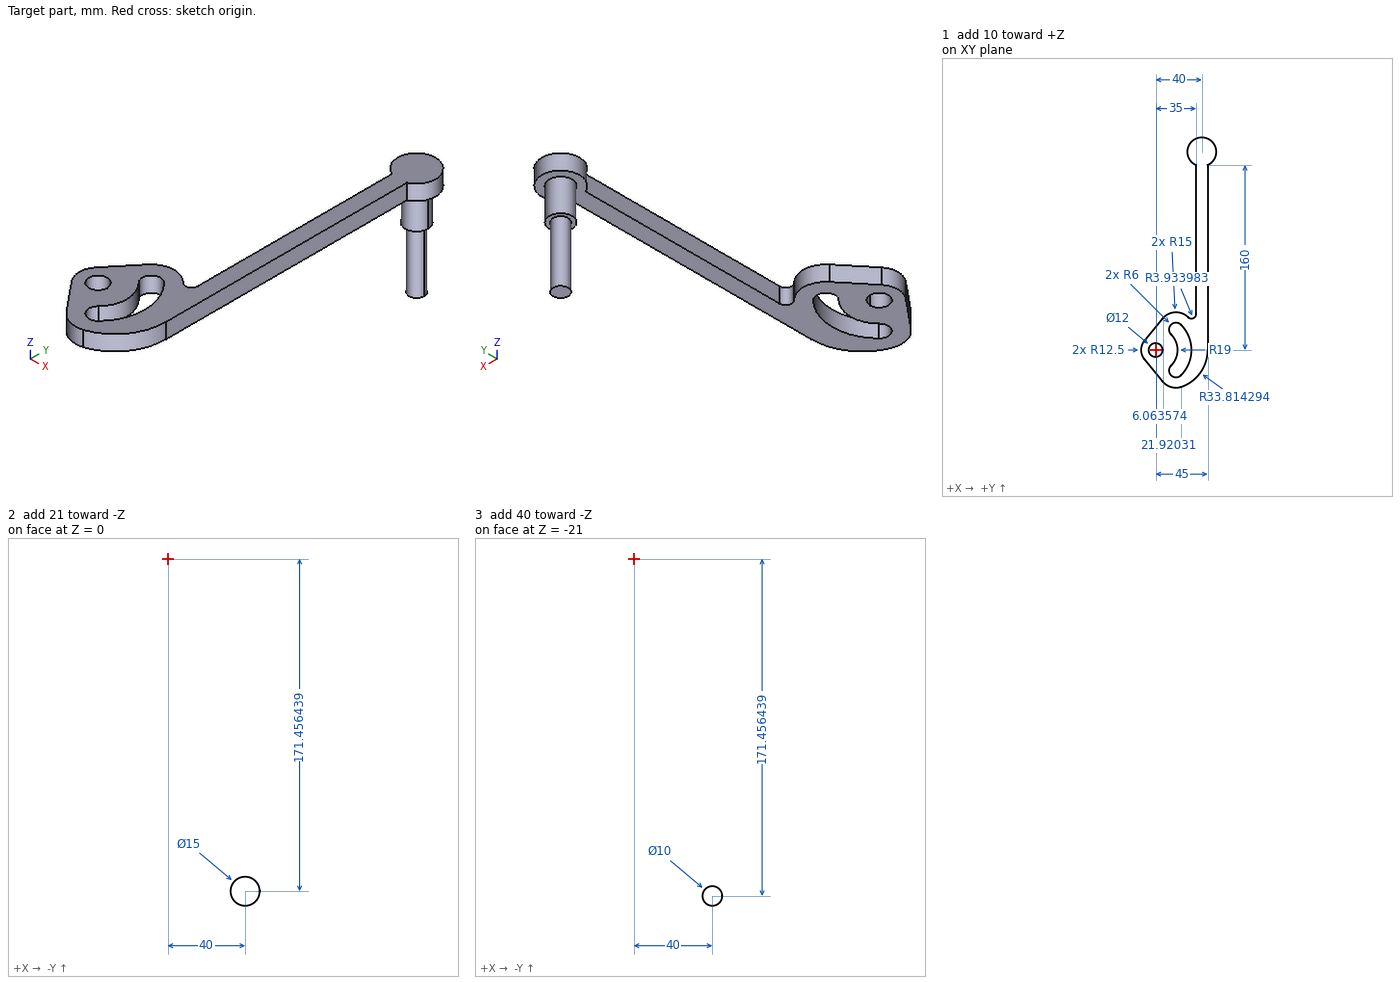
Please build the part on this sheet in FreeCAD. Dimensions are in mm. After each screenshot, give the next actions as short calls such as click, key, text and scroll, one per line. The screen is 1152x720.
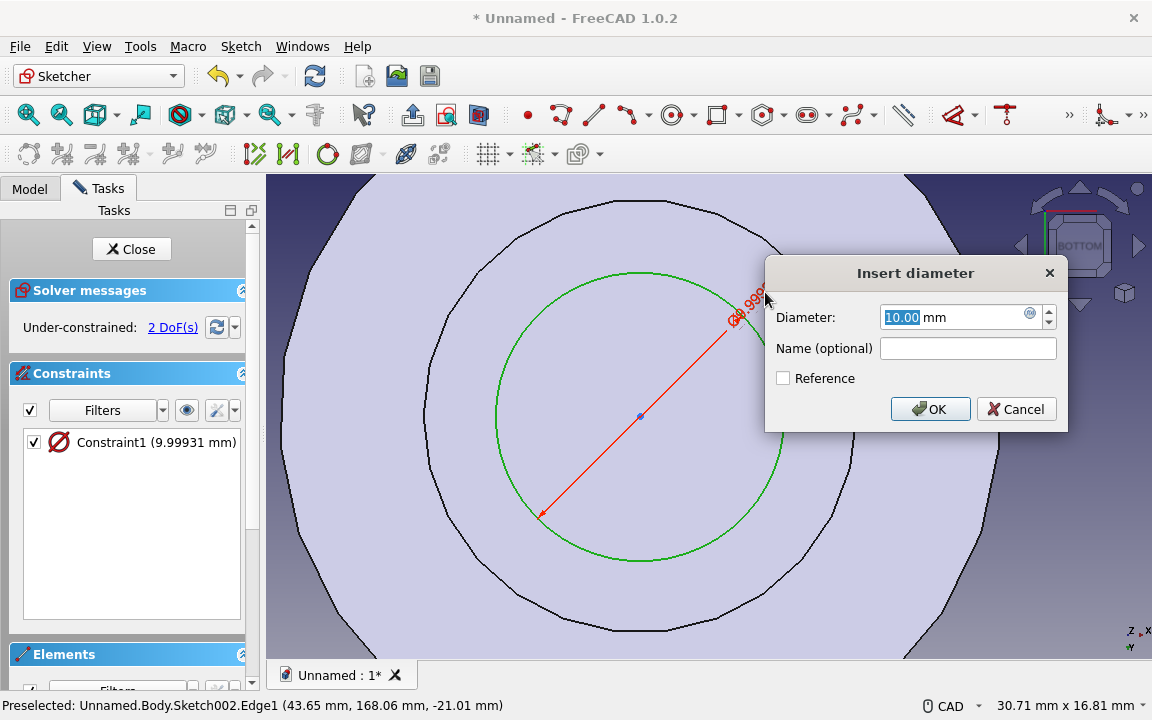
text(10)
key(Return)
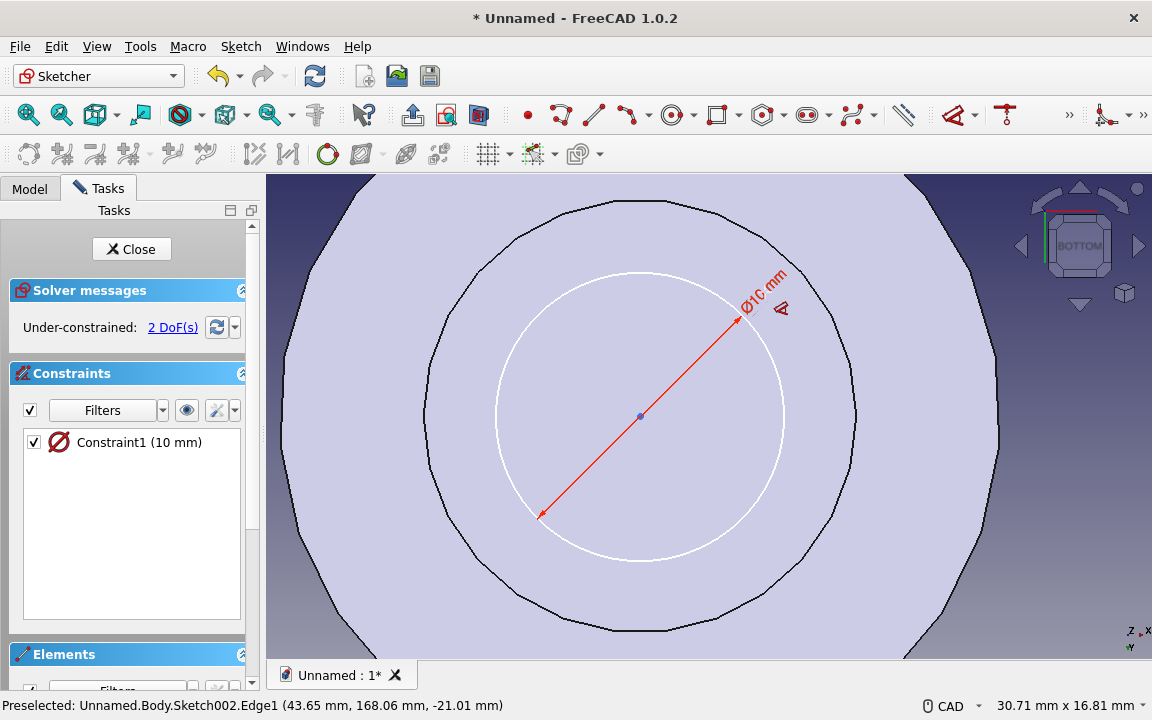
click(640, 417)
click(467, 451)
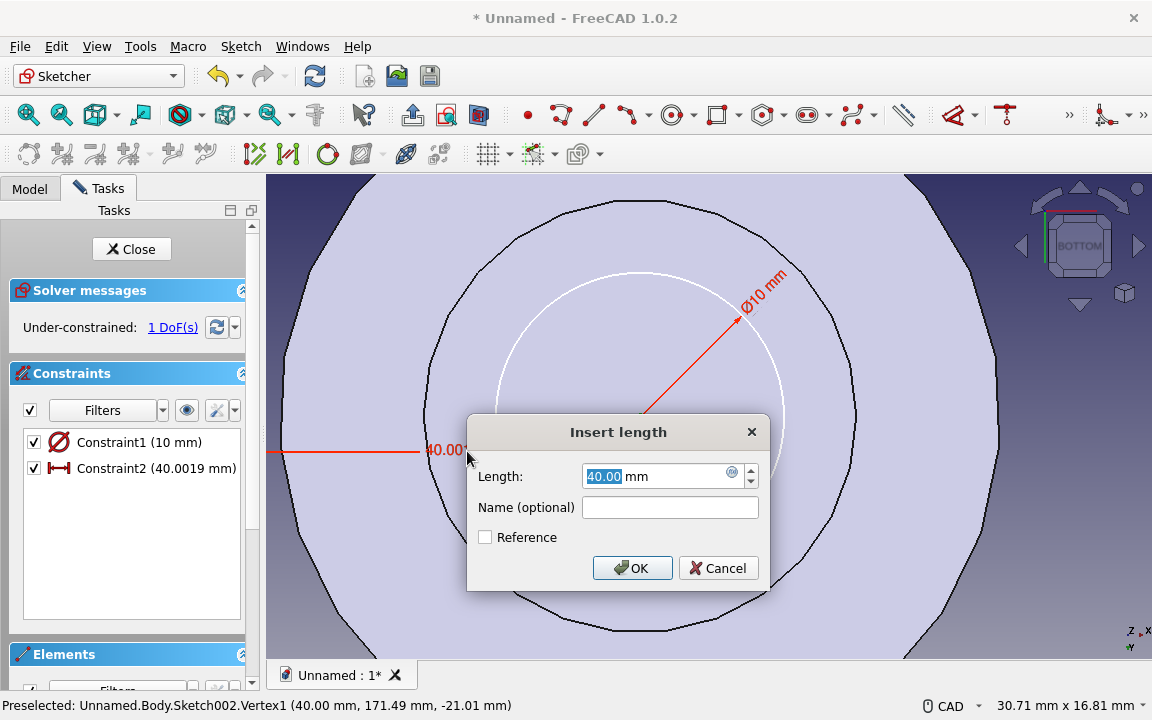
text(40)
key(Return)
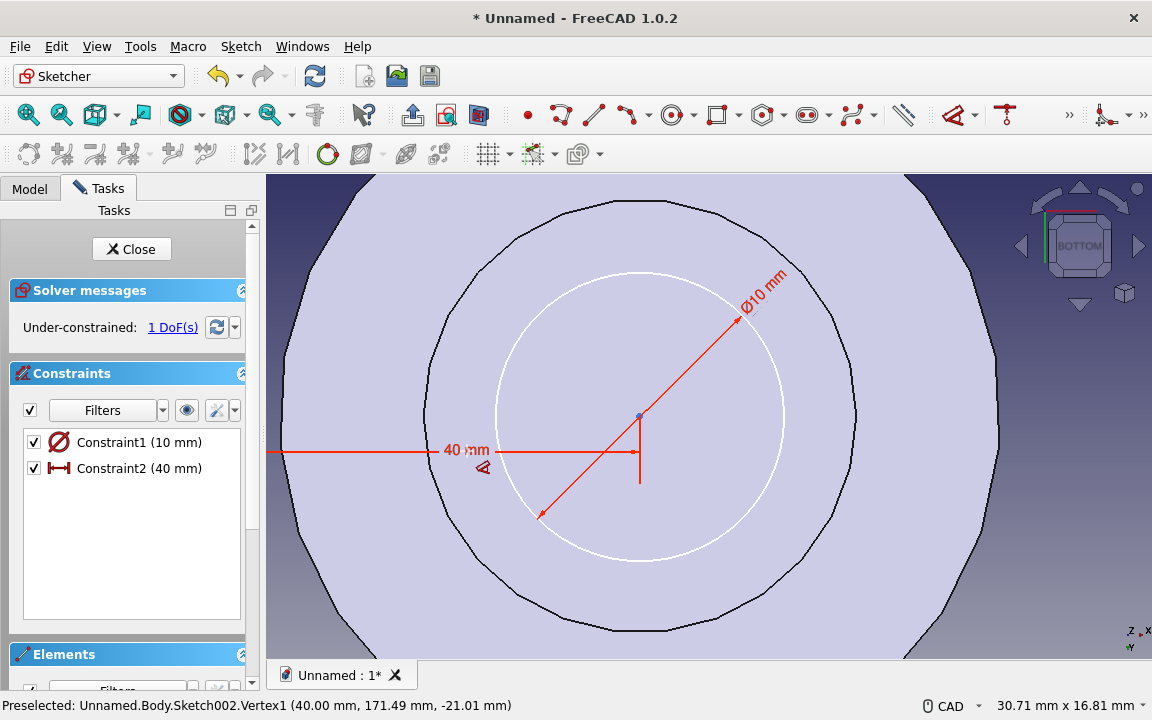
click(640, 417)
click(674, 310)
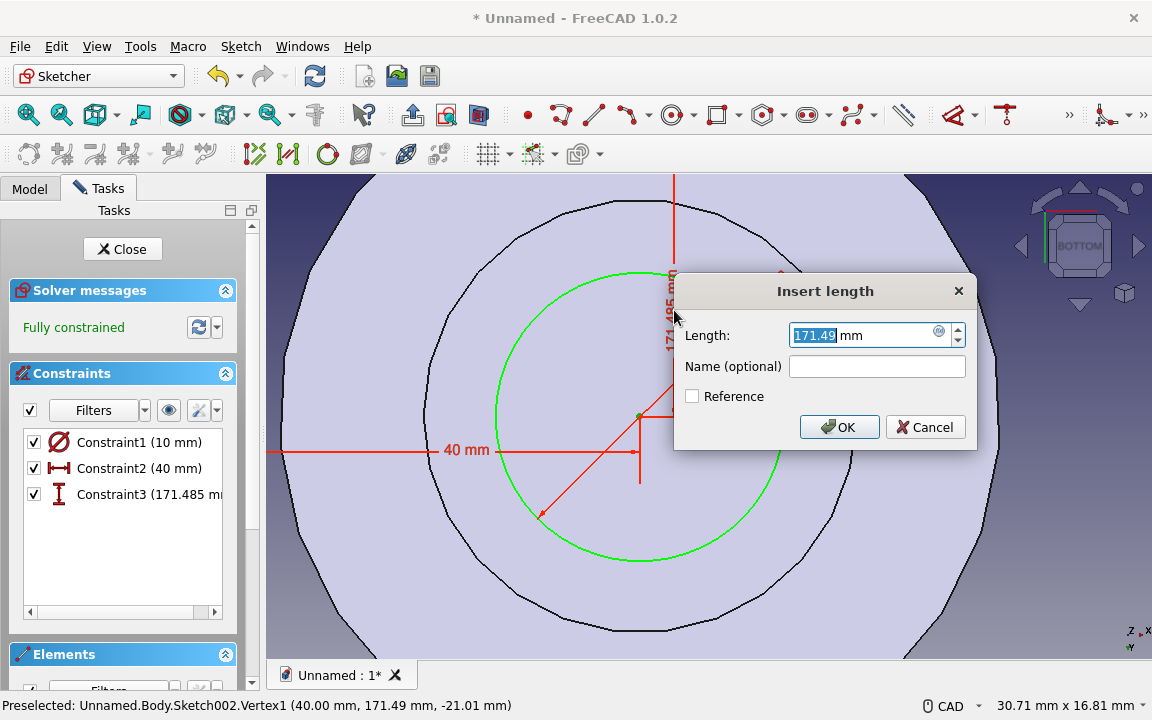
text(171.456439)
key(Return)
key(Escape)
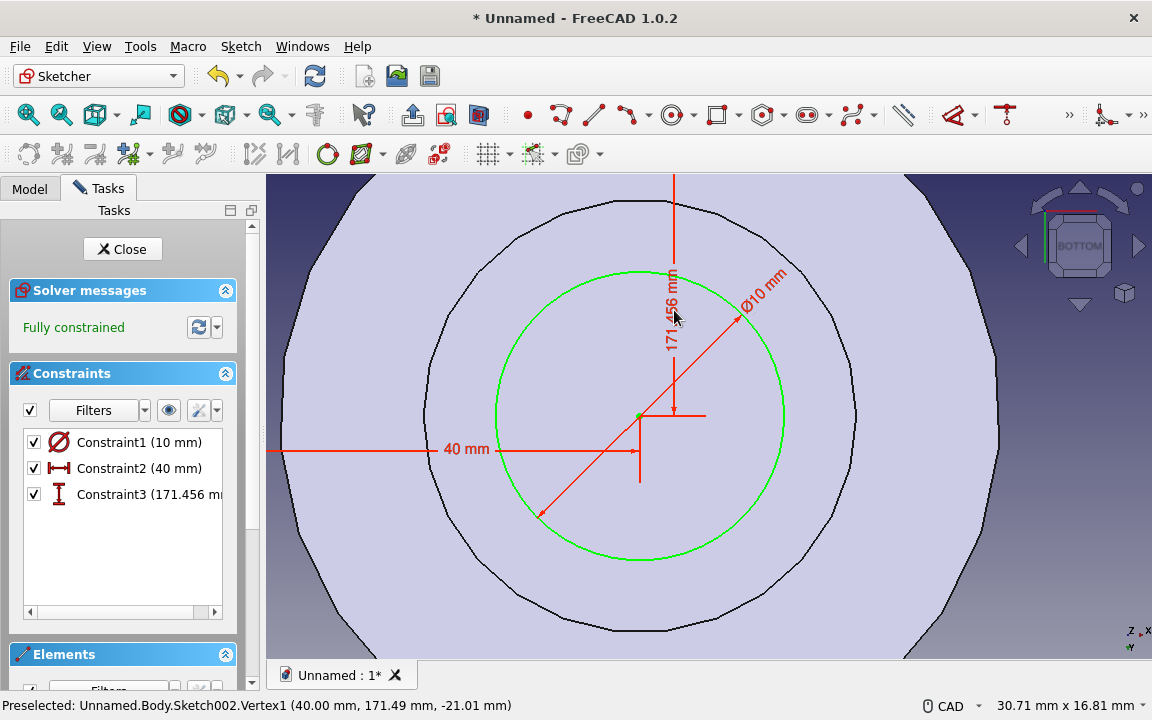
click(123, 249)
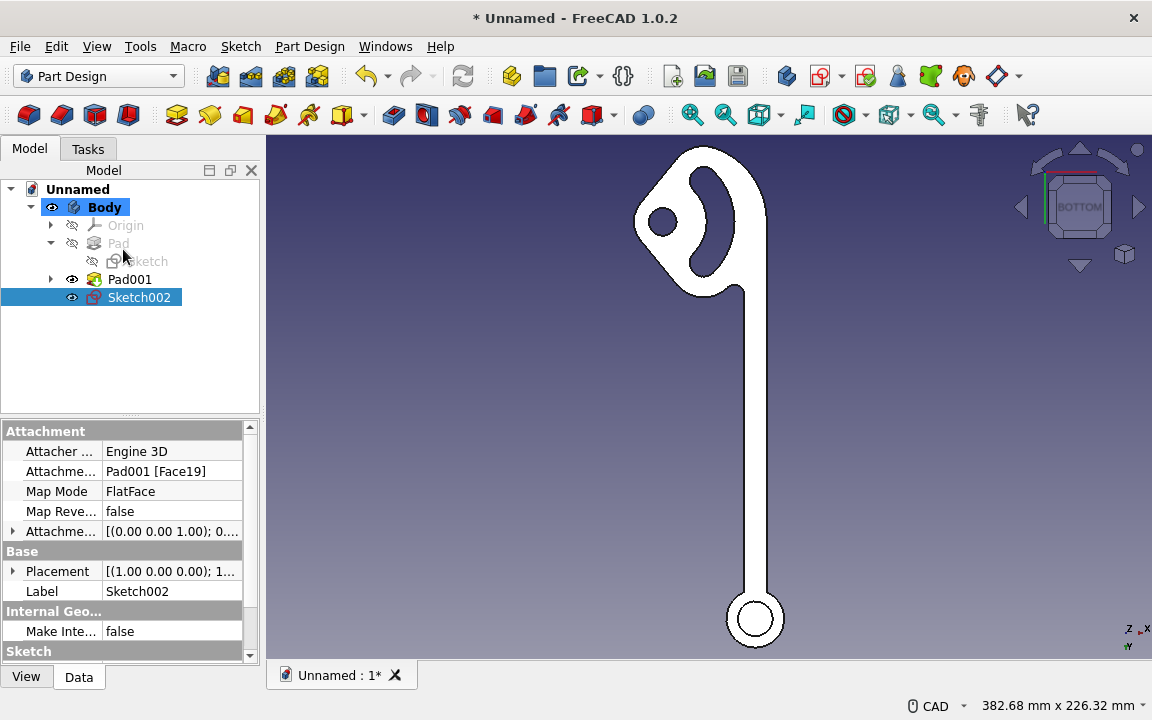
click(177, 116)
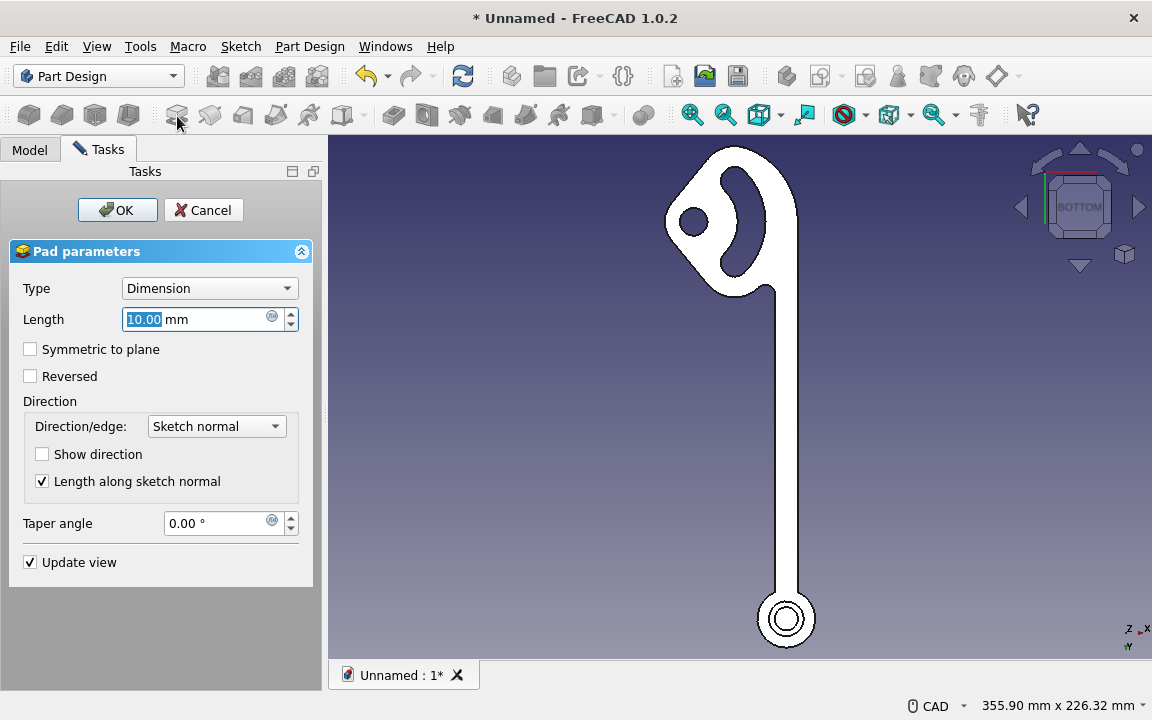
text(40)
key(Tab)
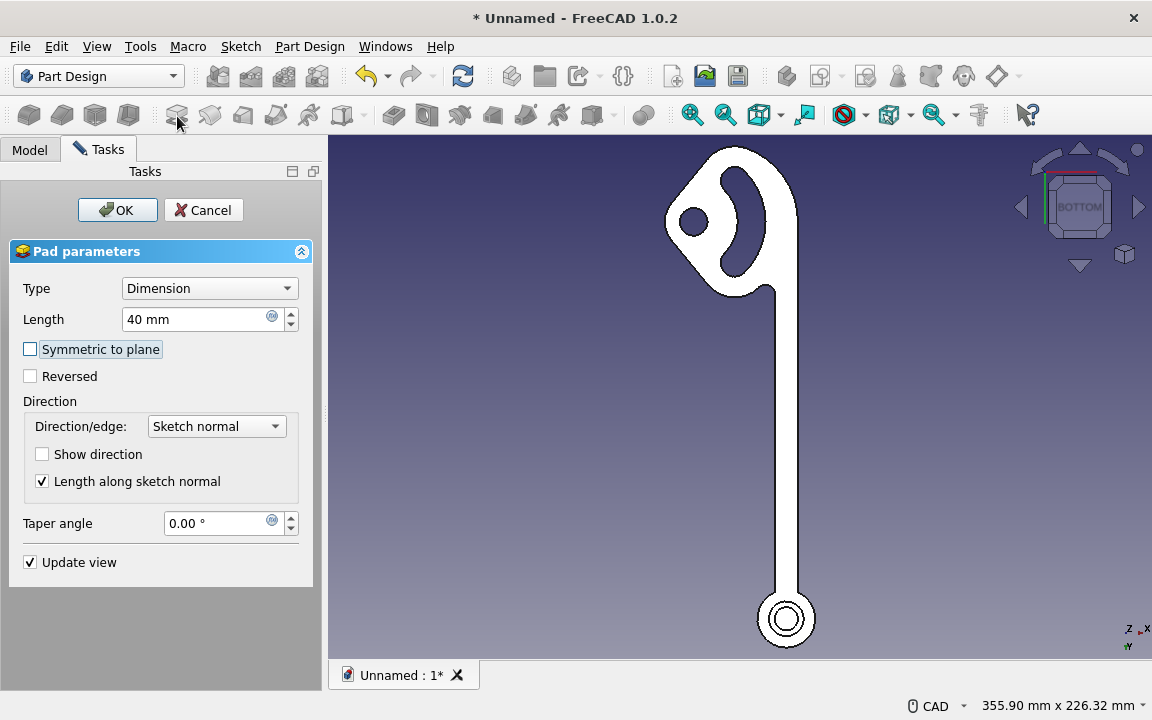
click(118, 210)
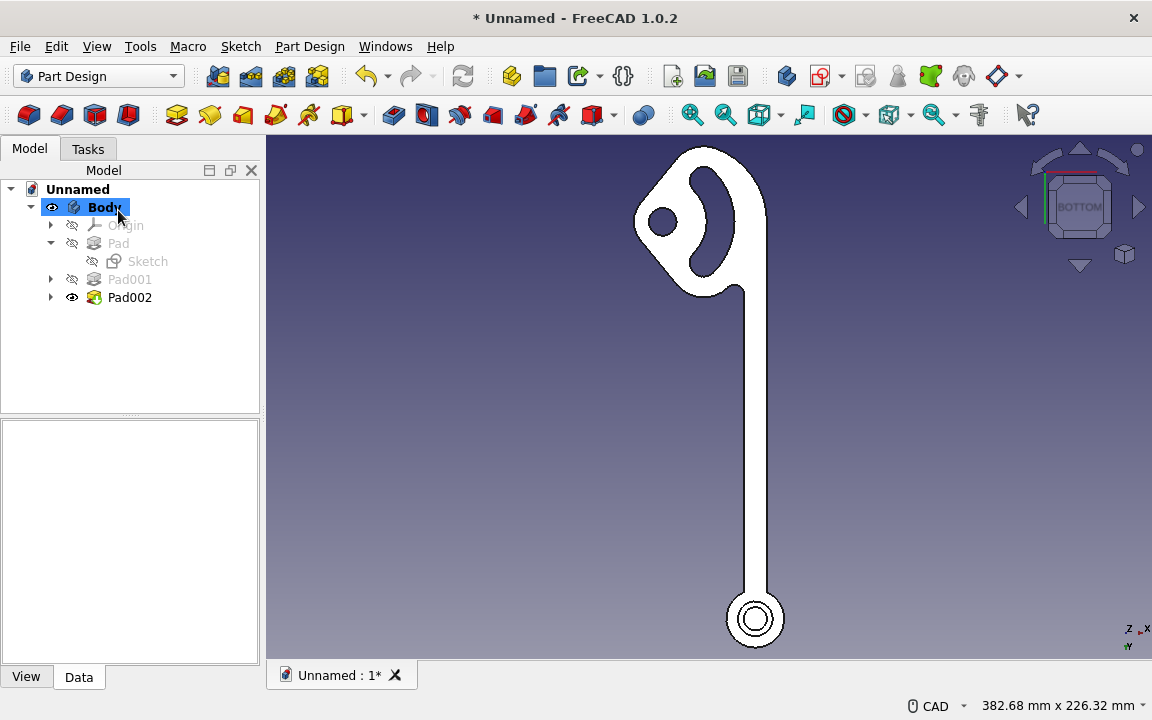
key(0)